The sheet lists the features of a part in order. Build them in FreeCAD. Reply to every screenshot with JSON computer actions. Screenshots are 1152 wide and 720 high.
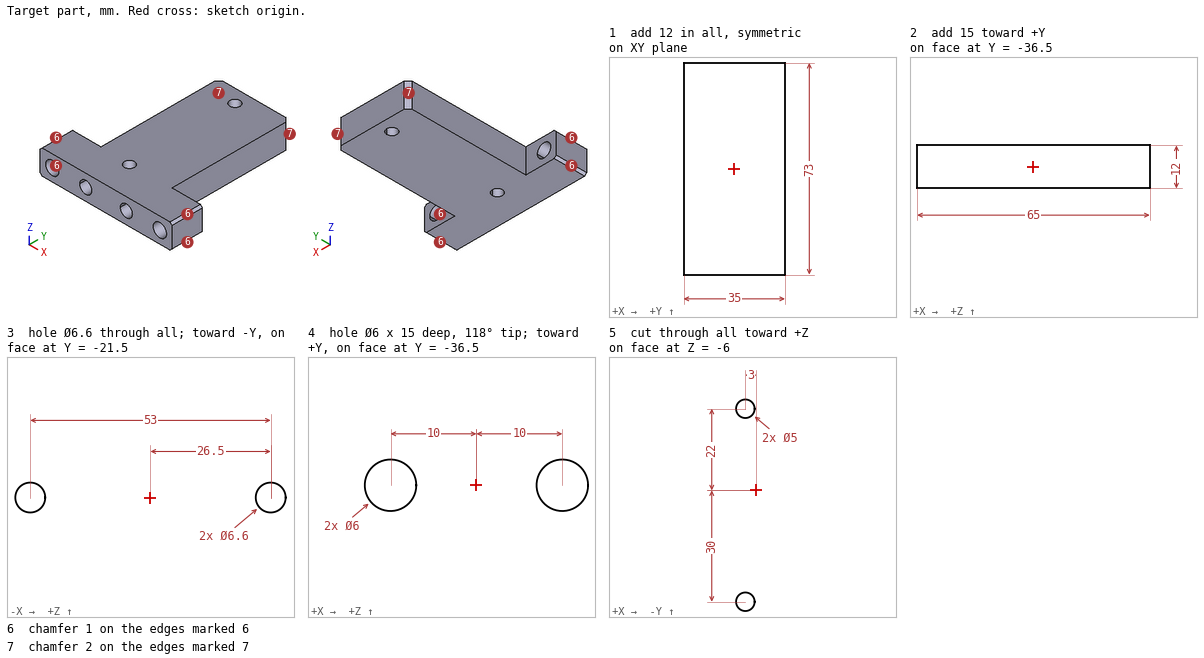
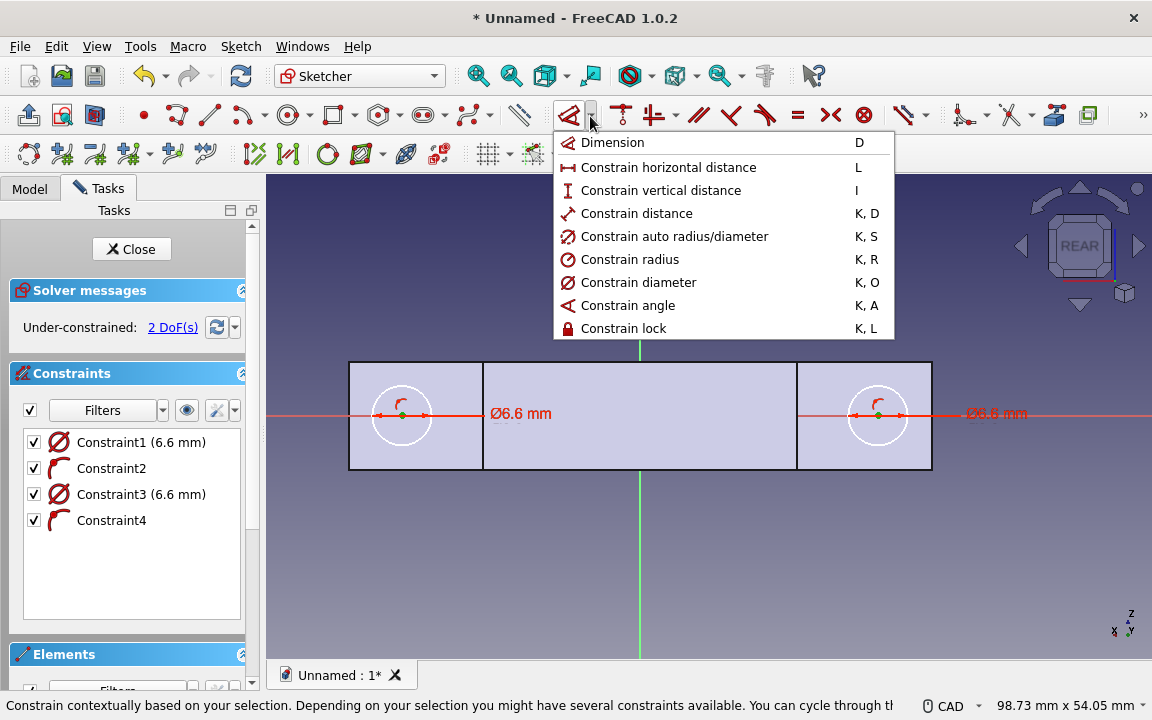
{"action": "left_click", "coordinate": [724, 168]}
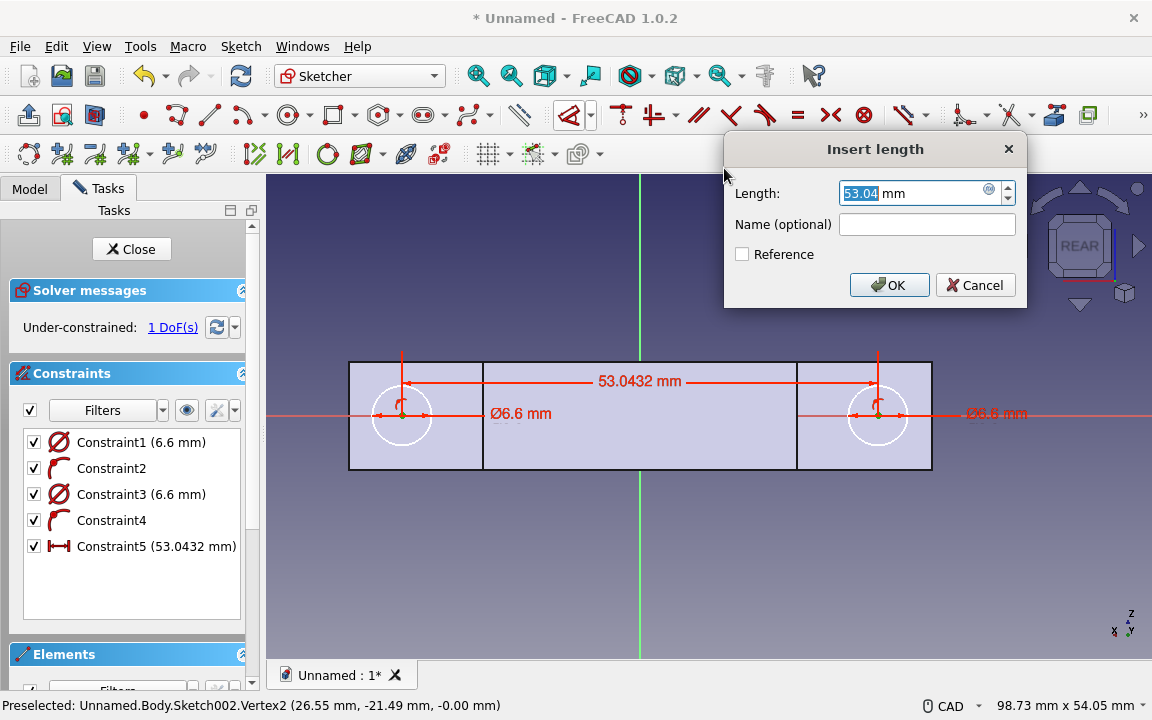
{"action": "type", "text": "53"}
{"action": "key", "text": "Return"}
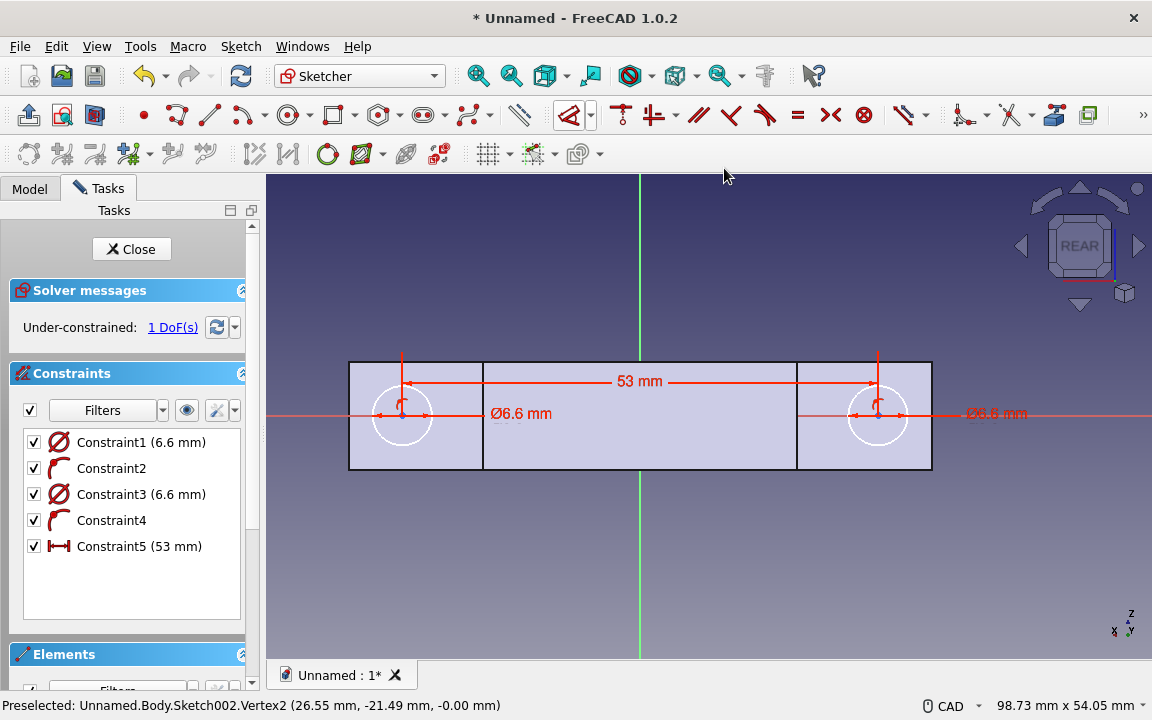
{"action": "left_click", "coordinate": [878, 416]}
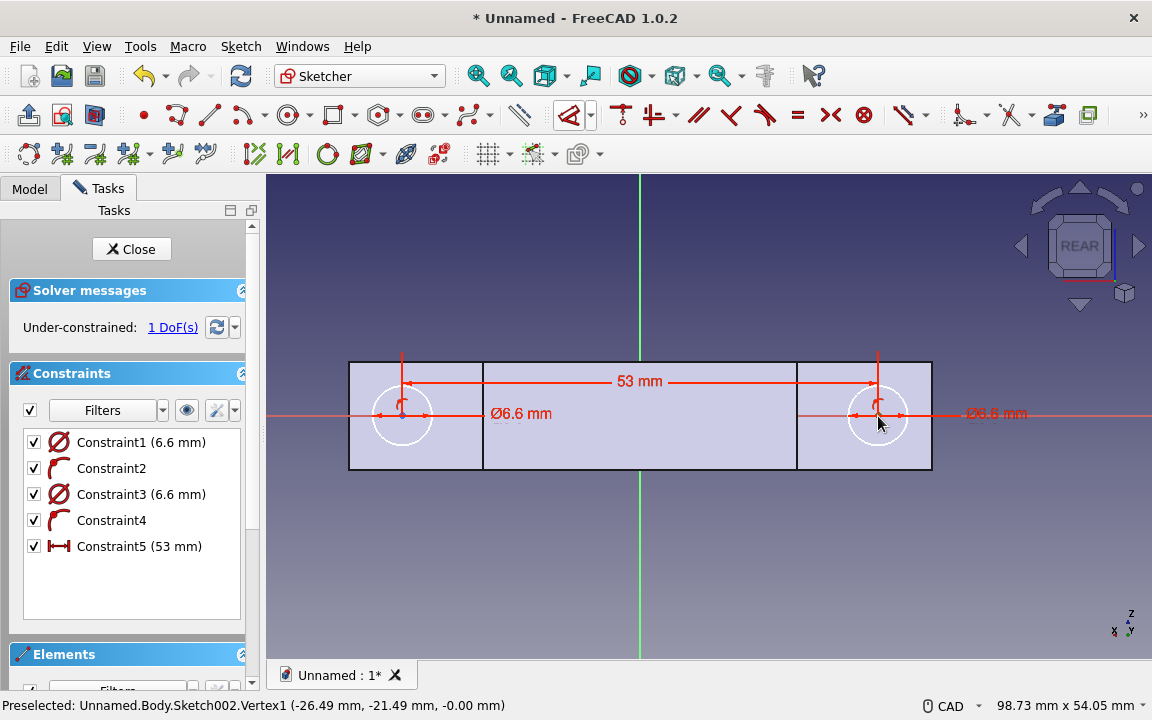
{"action": "left_click", "coordinate": [590, 116]}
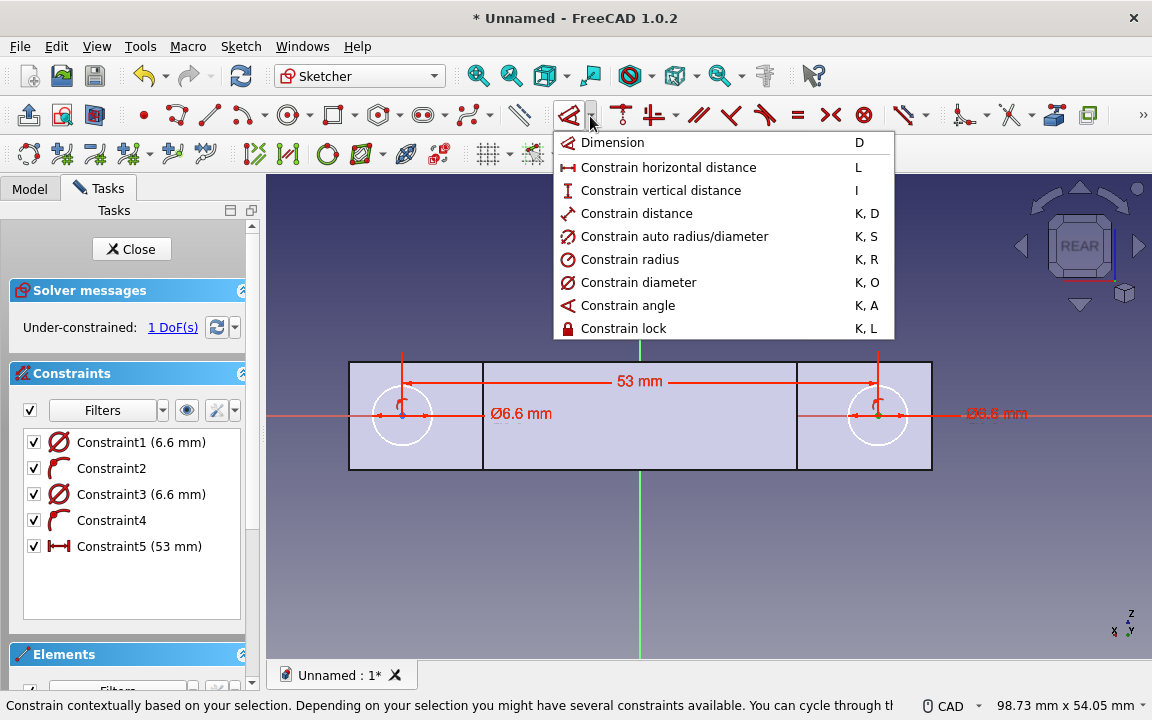
{"action": "left_click", "coordinate": [724, 168]}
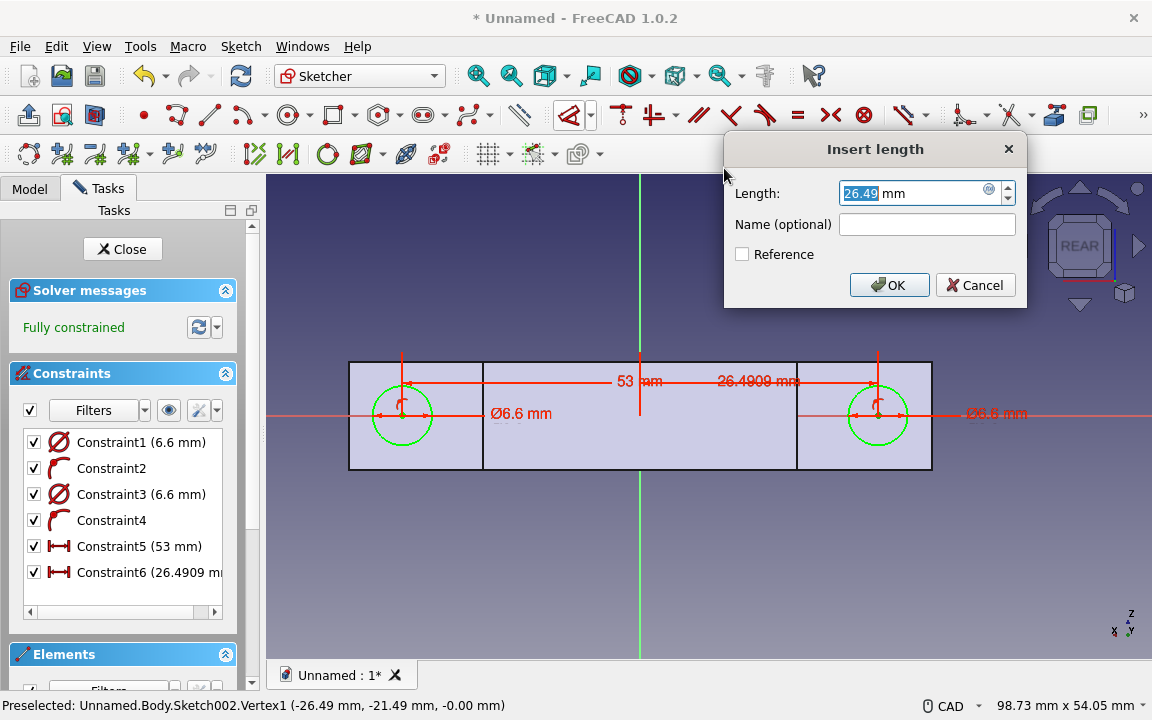
{"action": "type", "text": "26.5"}
{"action": "key", "text": "Return"}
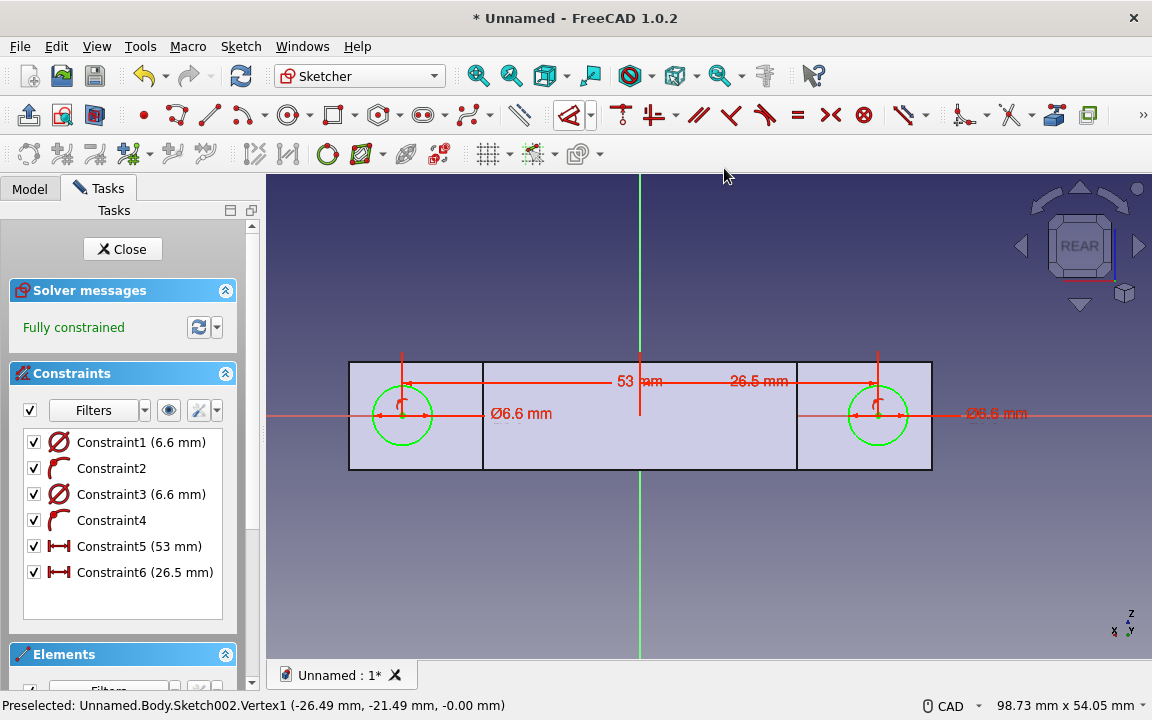
{"action": "left_click", "coordinate": [123, 249]}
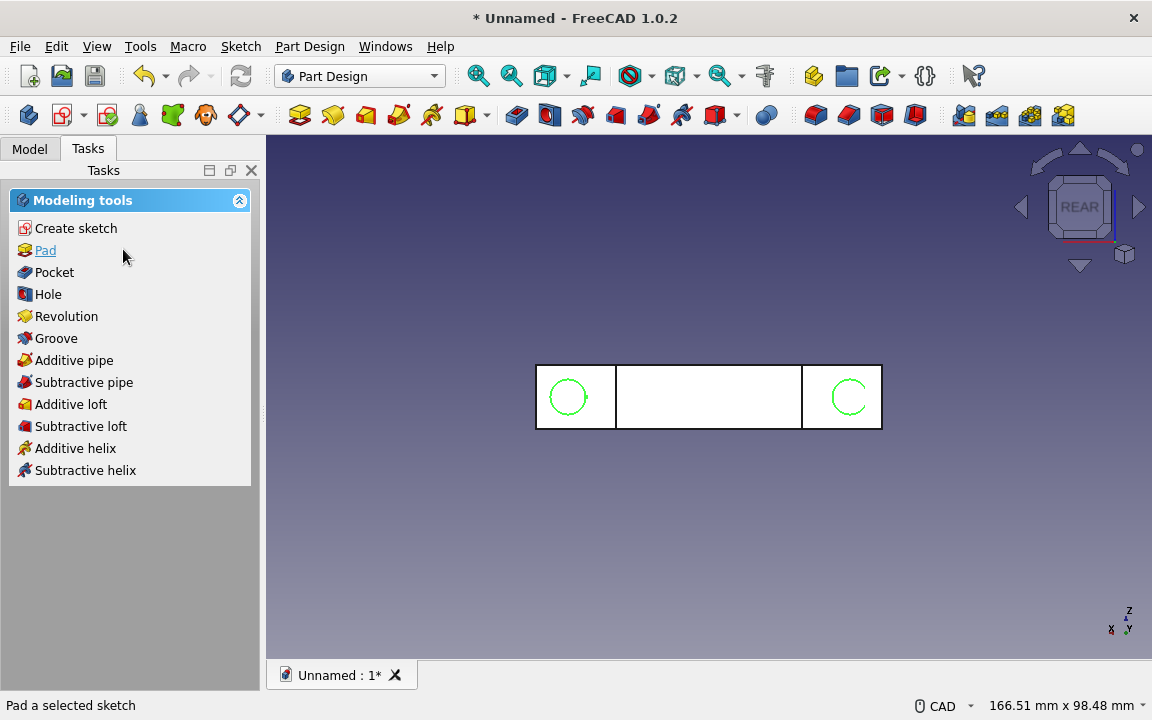
{"action": "left_click", "coordinate": [550, 116]}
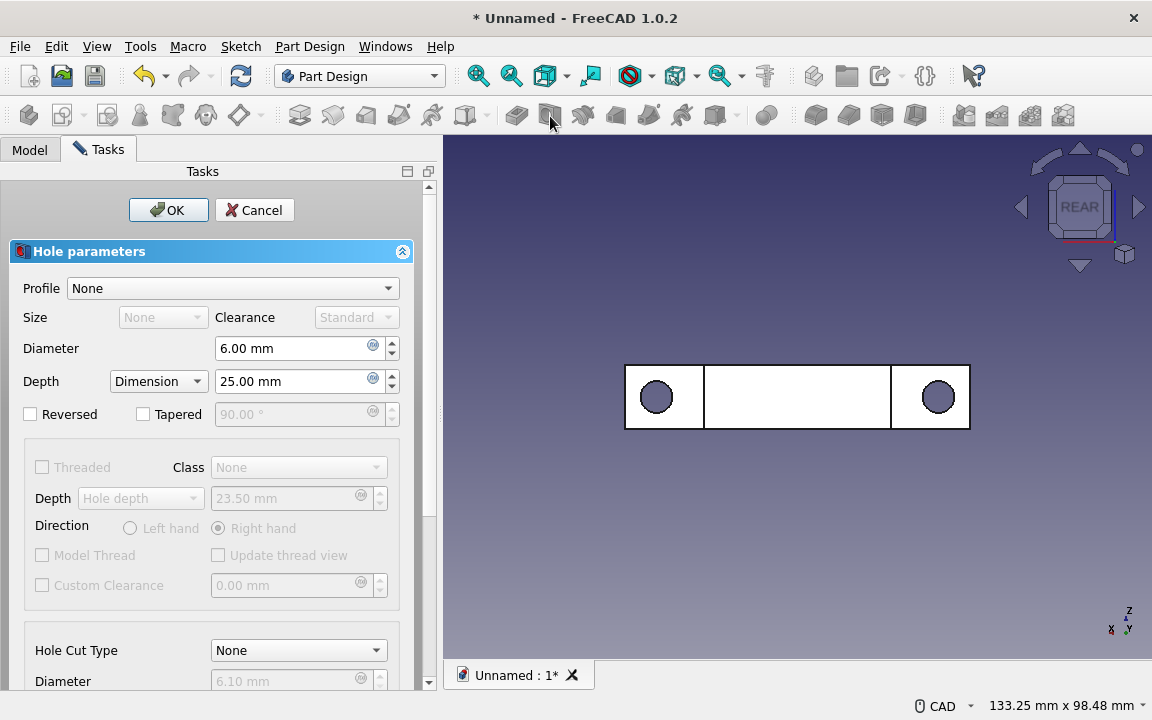
{"action": "triple_click", "coordinate": [300, 348]}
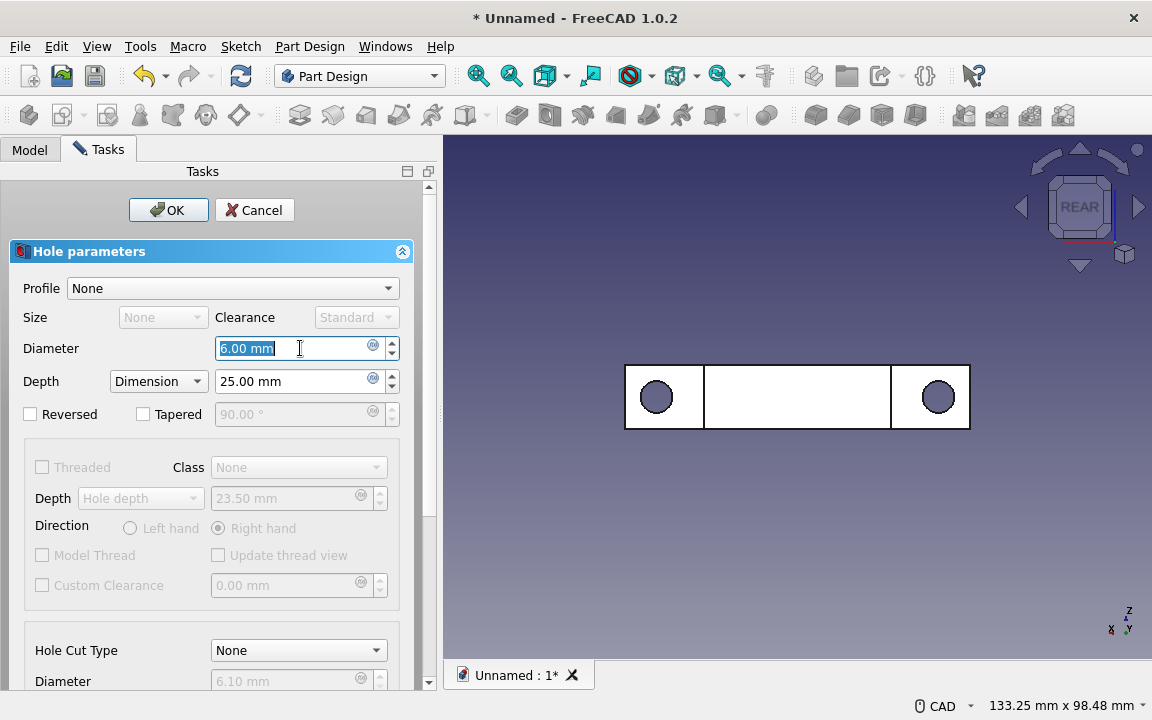
{"action": "type", "text": "6.6"}
{"action": "key", "text": "Tab"}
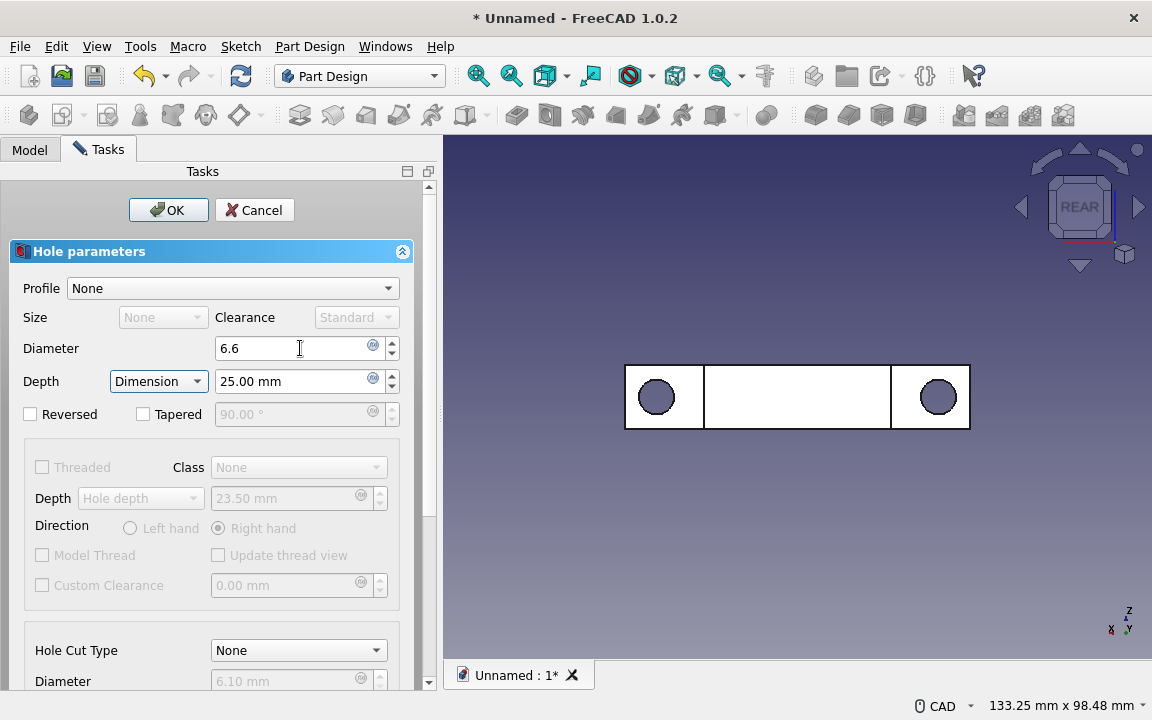
{"action": "left_click", "coordinate": [160, 382]}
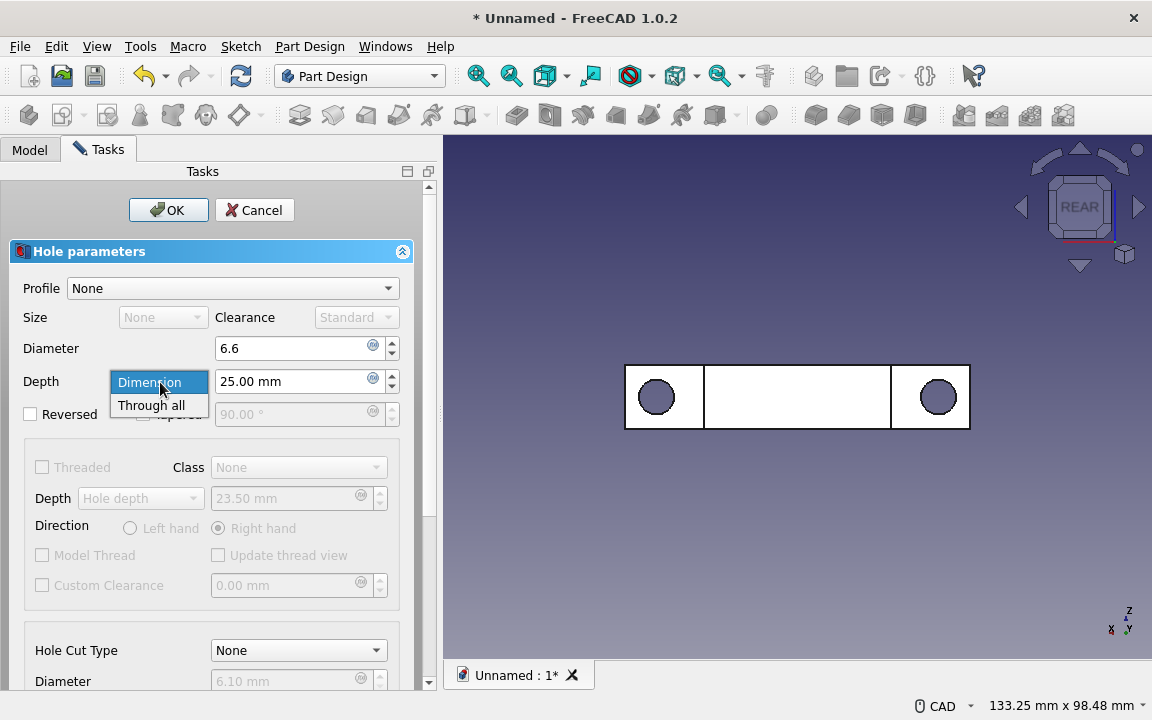
{"action": "left_click", "coordinate": [158, 406]}